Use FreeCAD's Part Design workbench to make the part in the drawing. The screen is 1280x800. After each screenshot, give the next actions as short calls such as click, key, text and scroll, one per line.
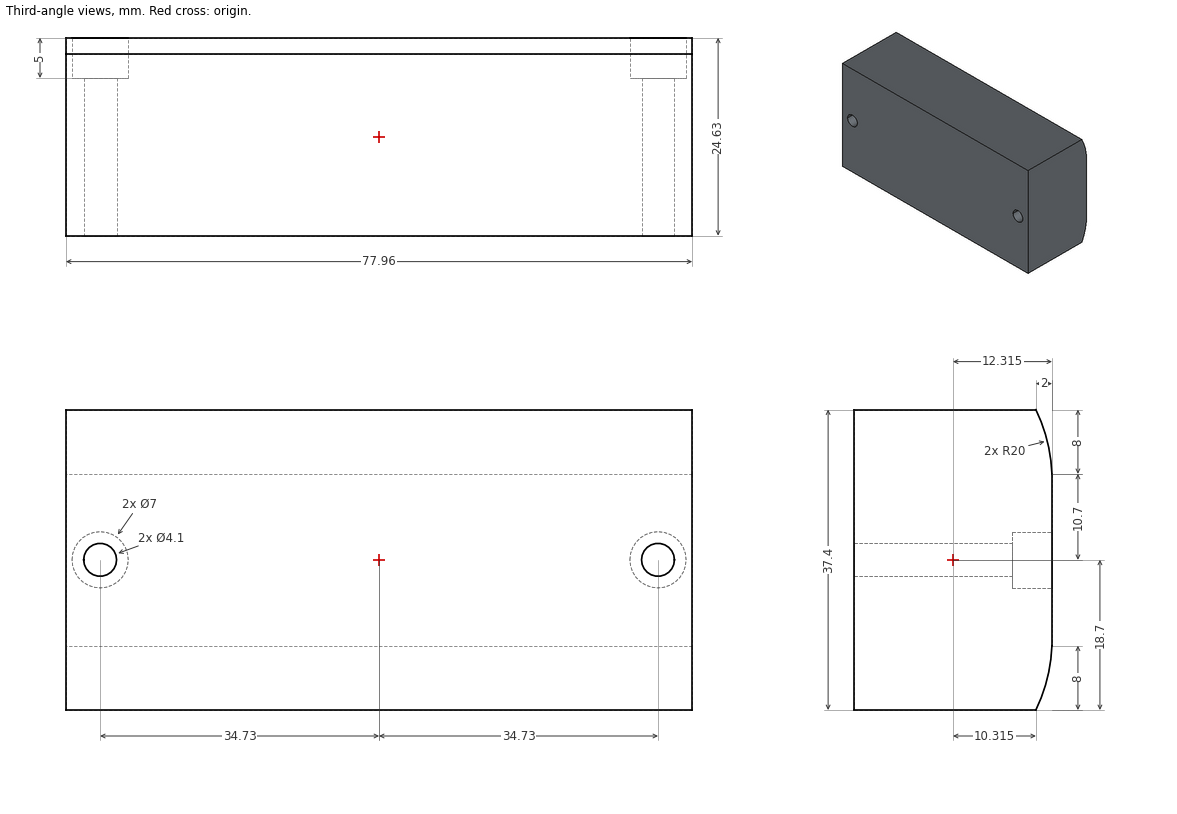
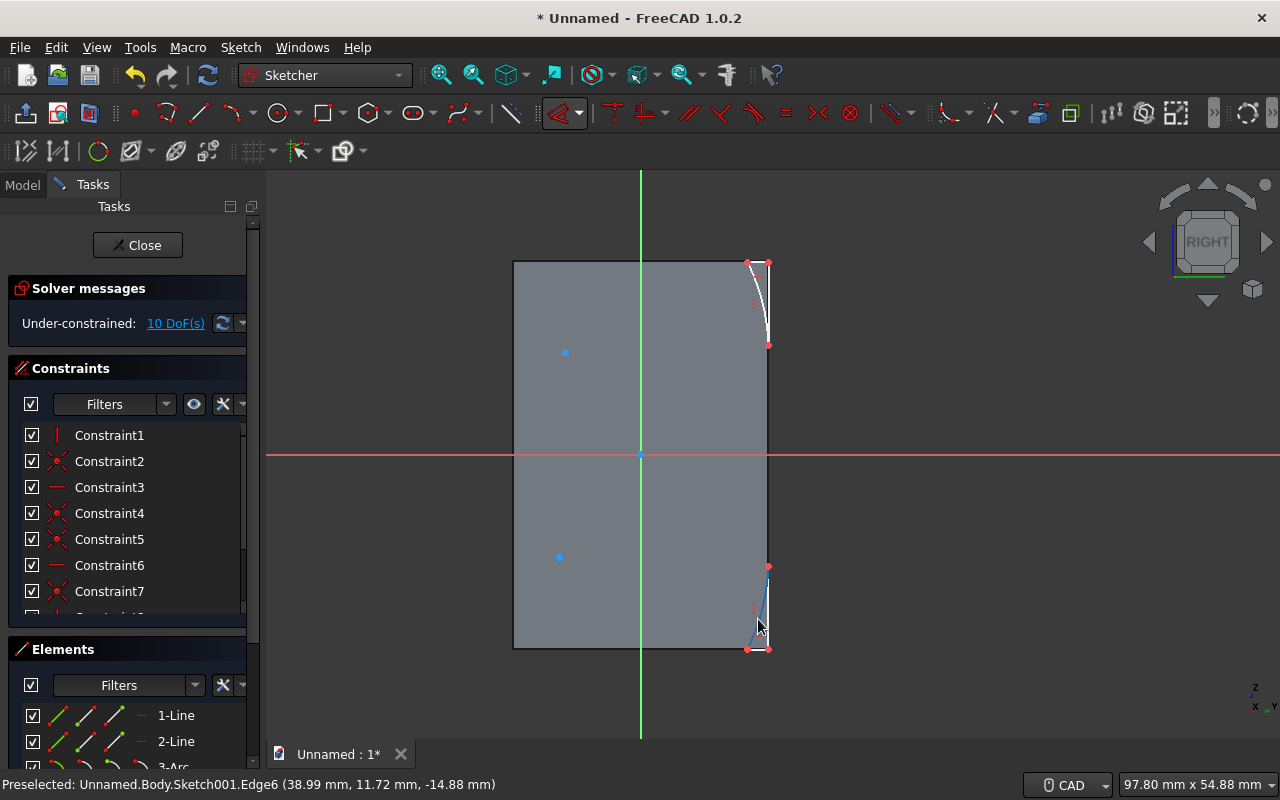
scroll(766, 320, up, 9)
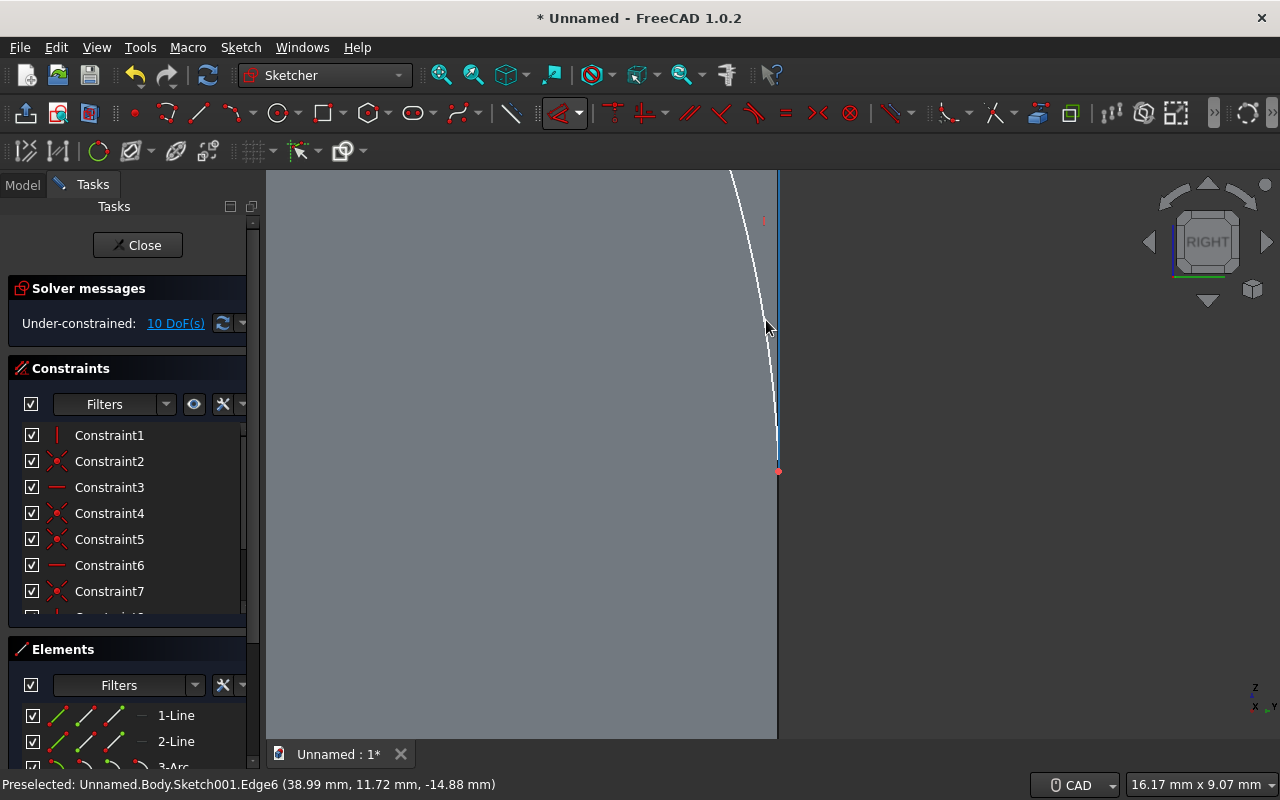
click(764, 316)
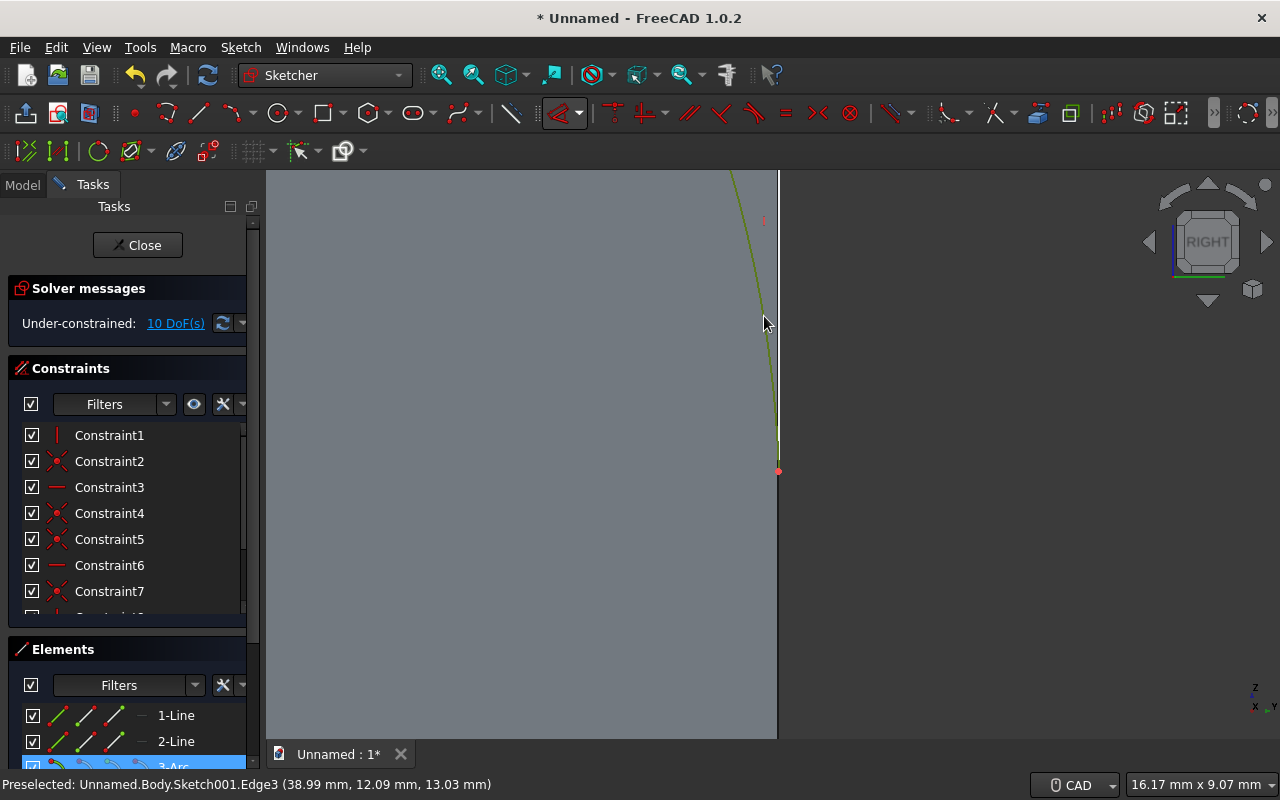
scroll(766, 320, down, 9)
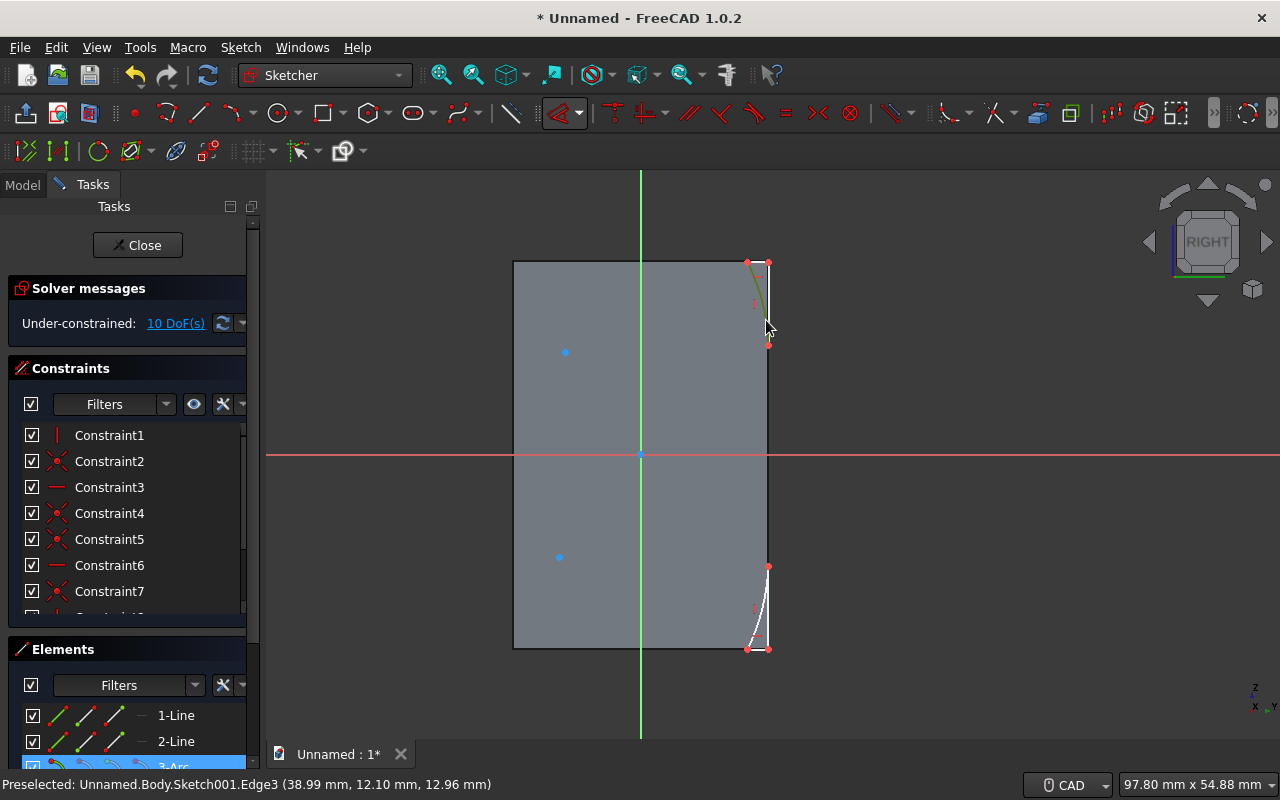
scroll(757, 626, up, 2)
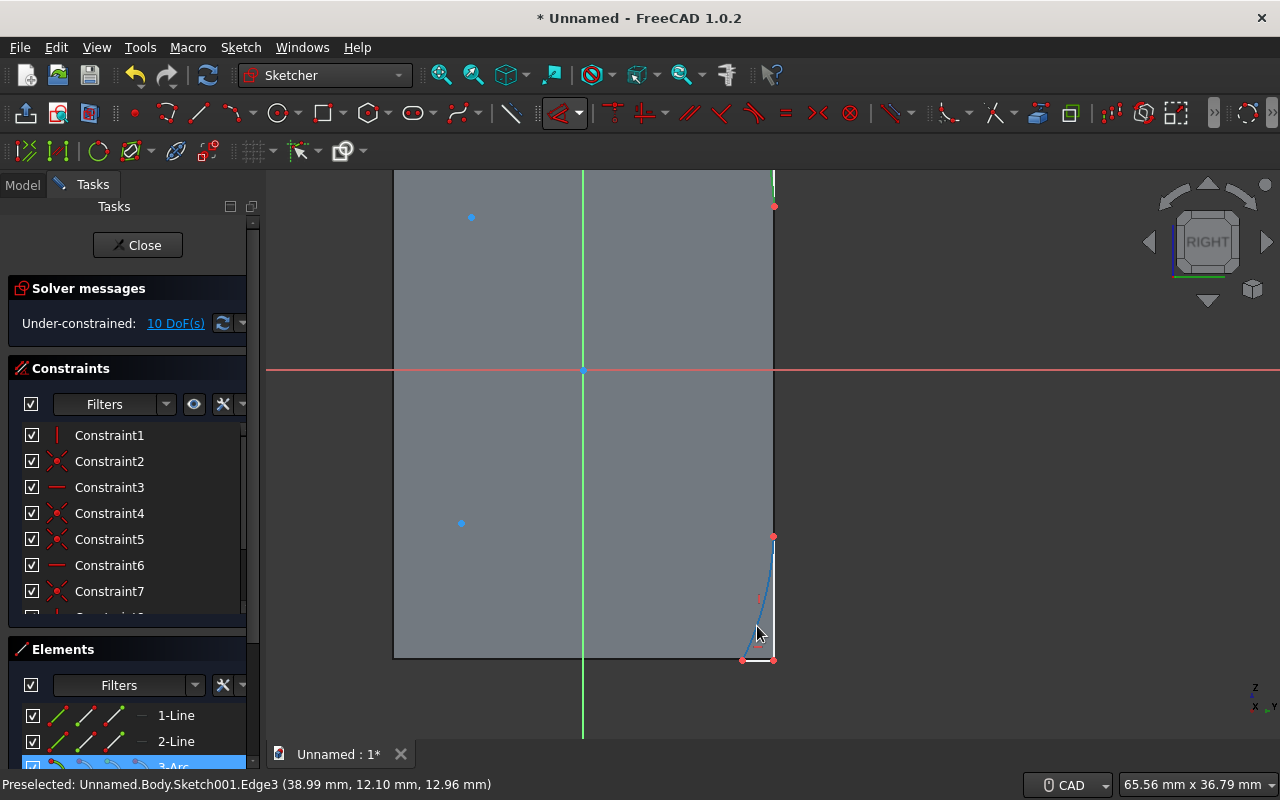
click(757, 625)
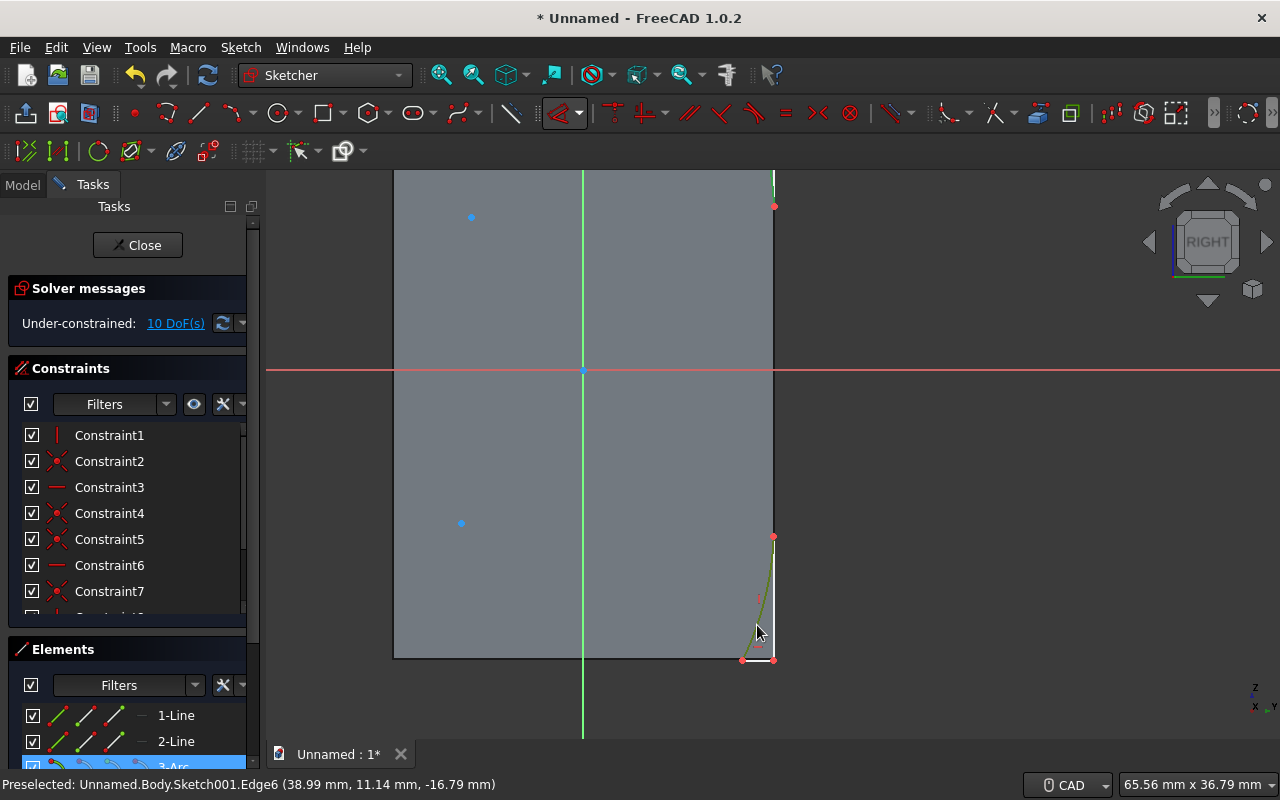
click(786, 114)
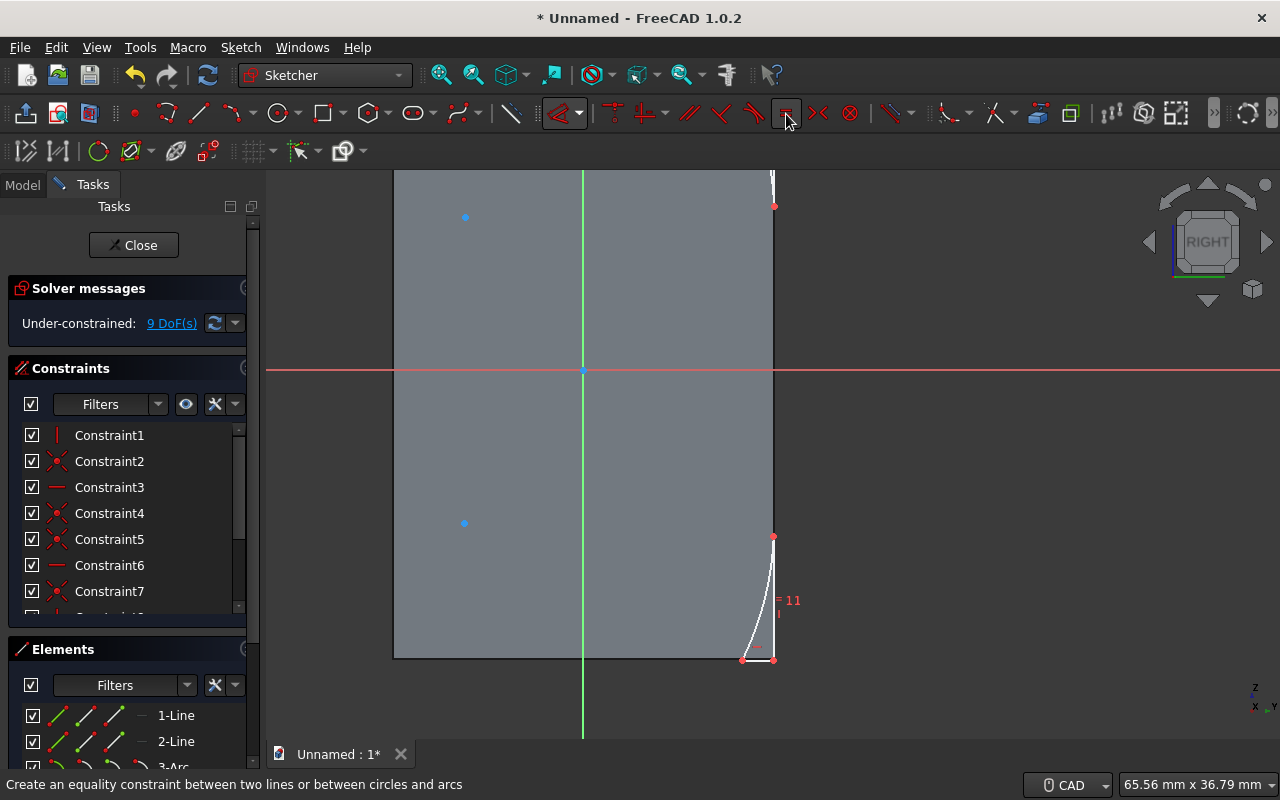
scroll(758, 626, down, 2)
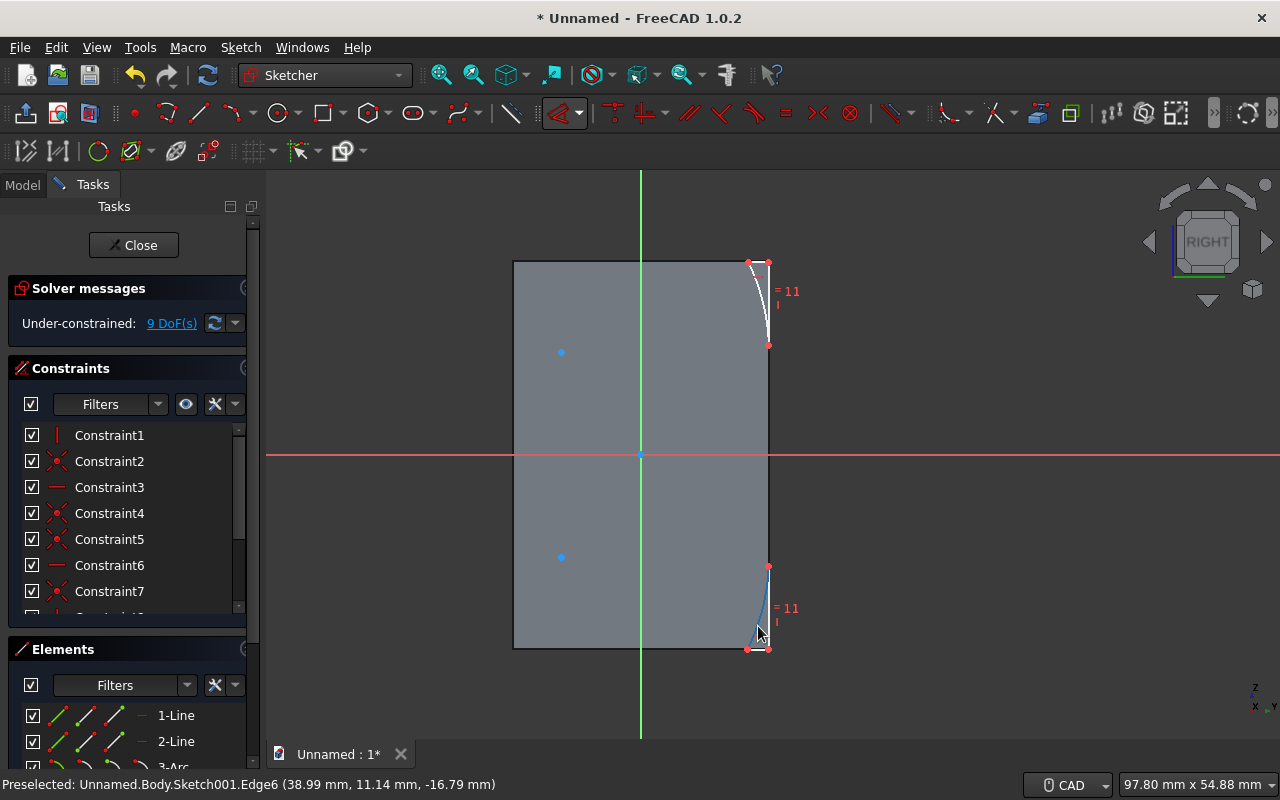
scroll(758, 286, up, 2)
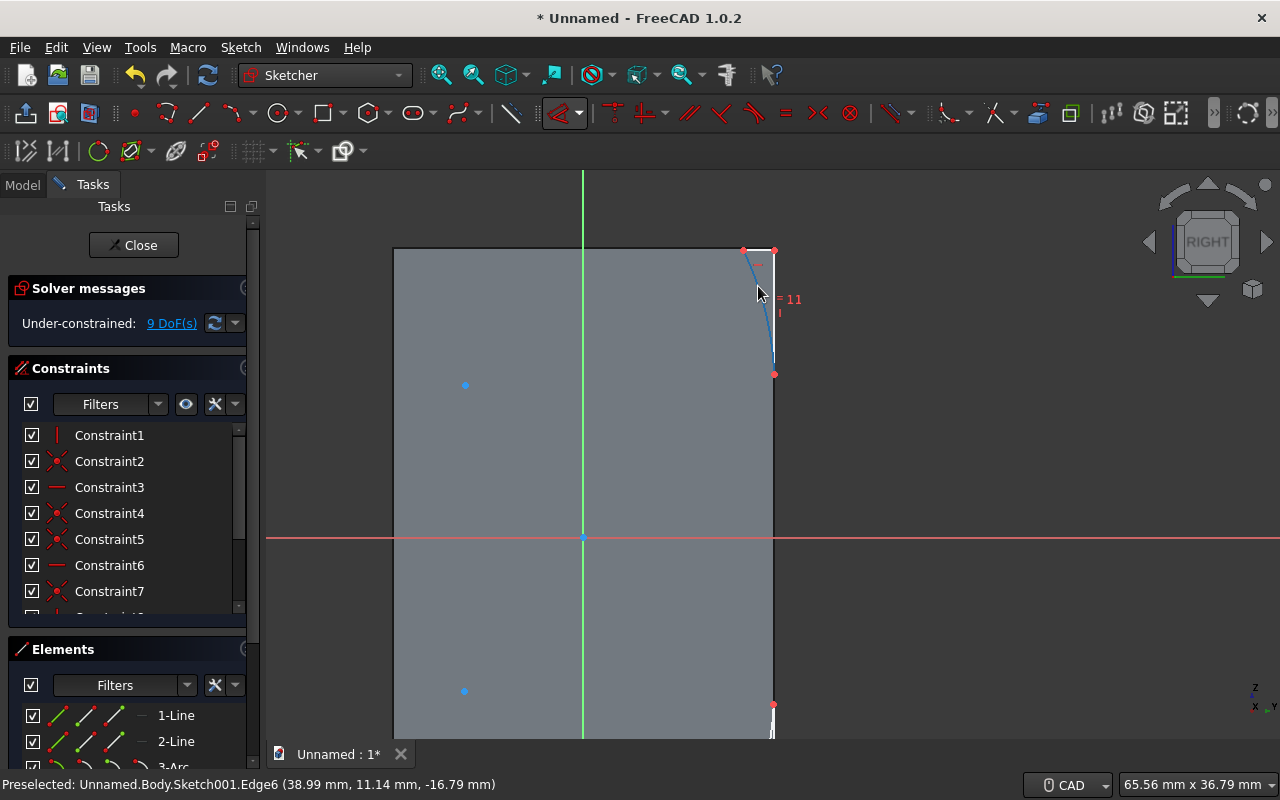
click(758, 286)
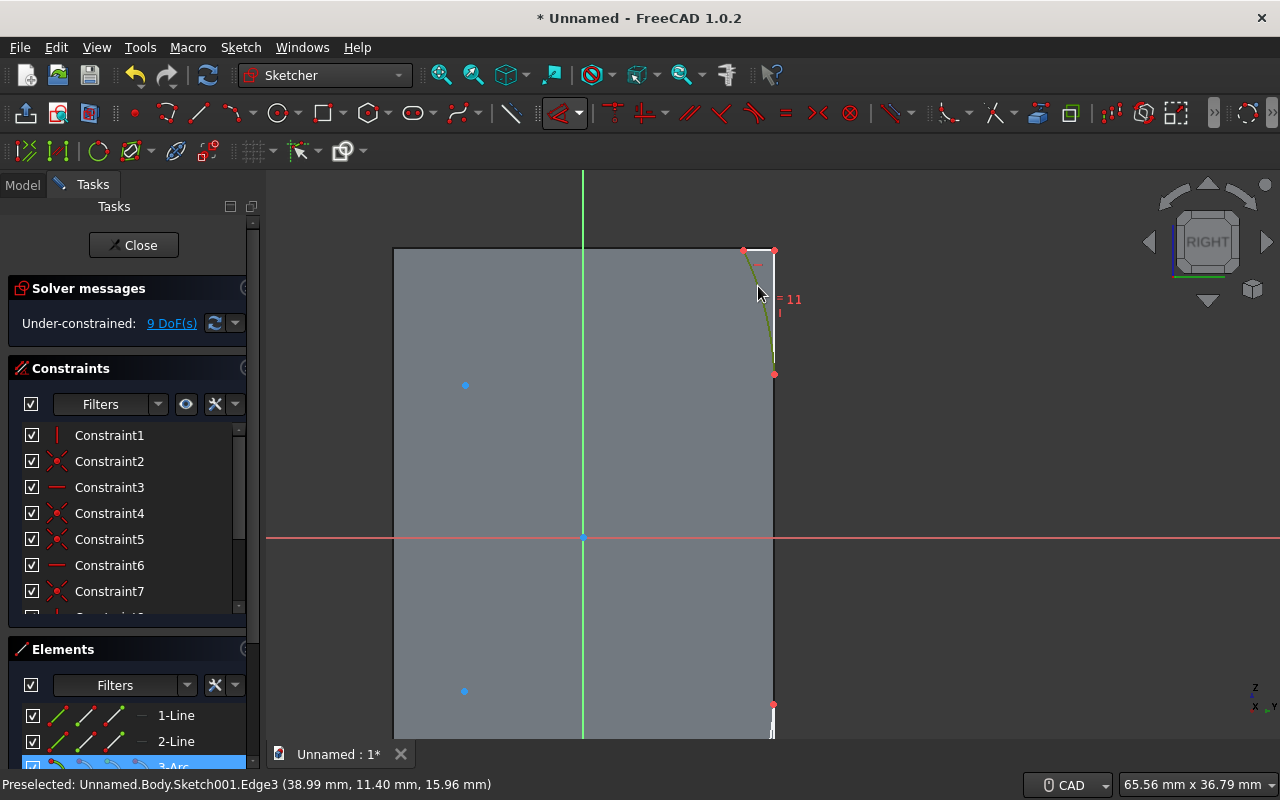
click(582, 114)